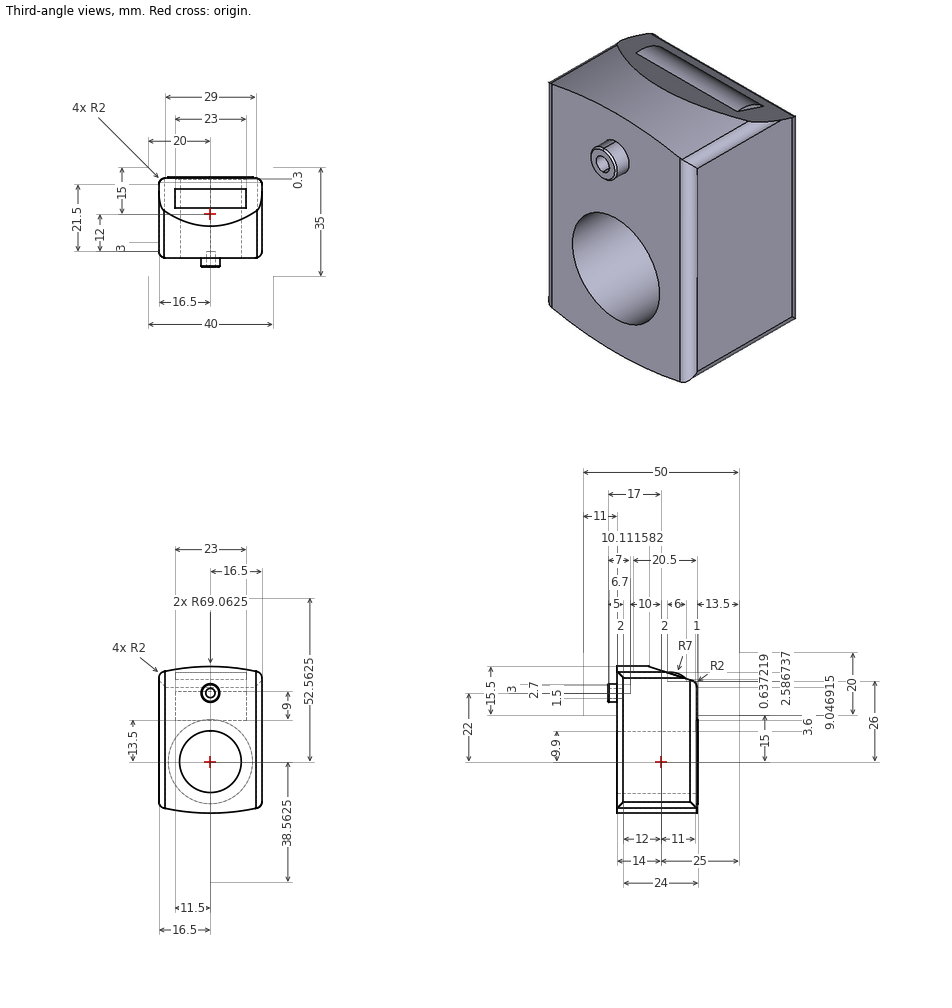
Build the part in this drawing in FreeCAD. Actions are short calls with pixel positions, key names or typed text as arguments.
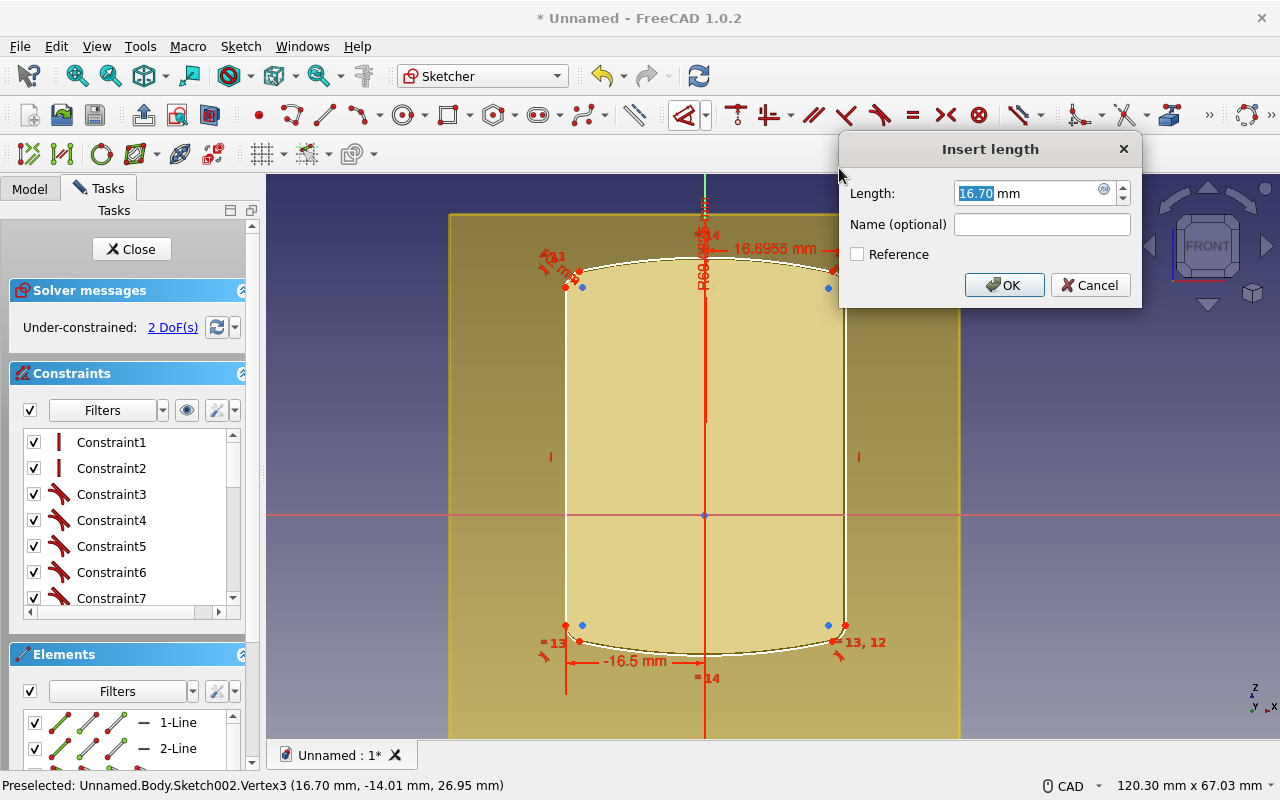
text(16.5)
key(Return)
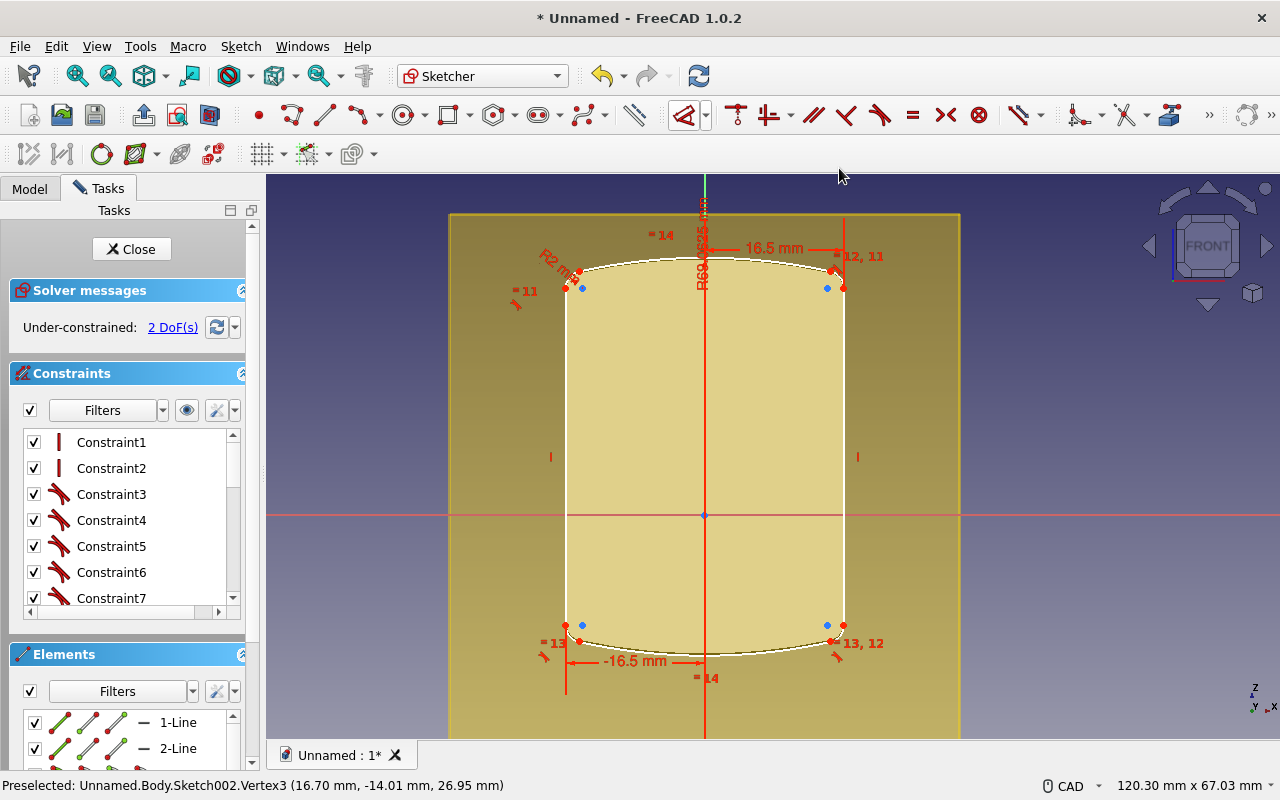
scroll(704, 268, down, 2)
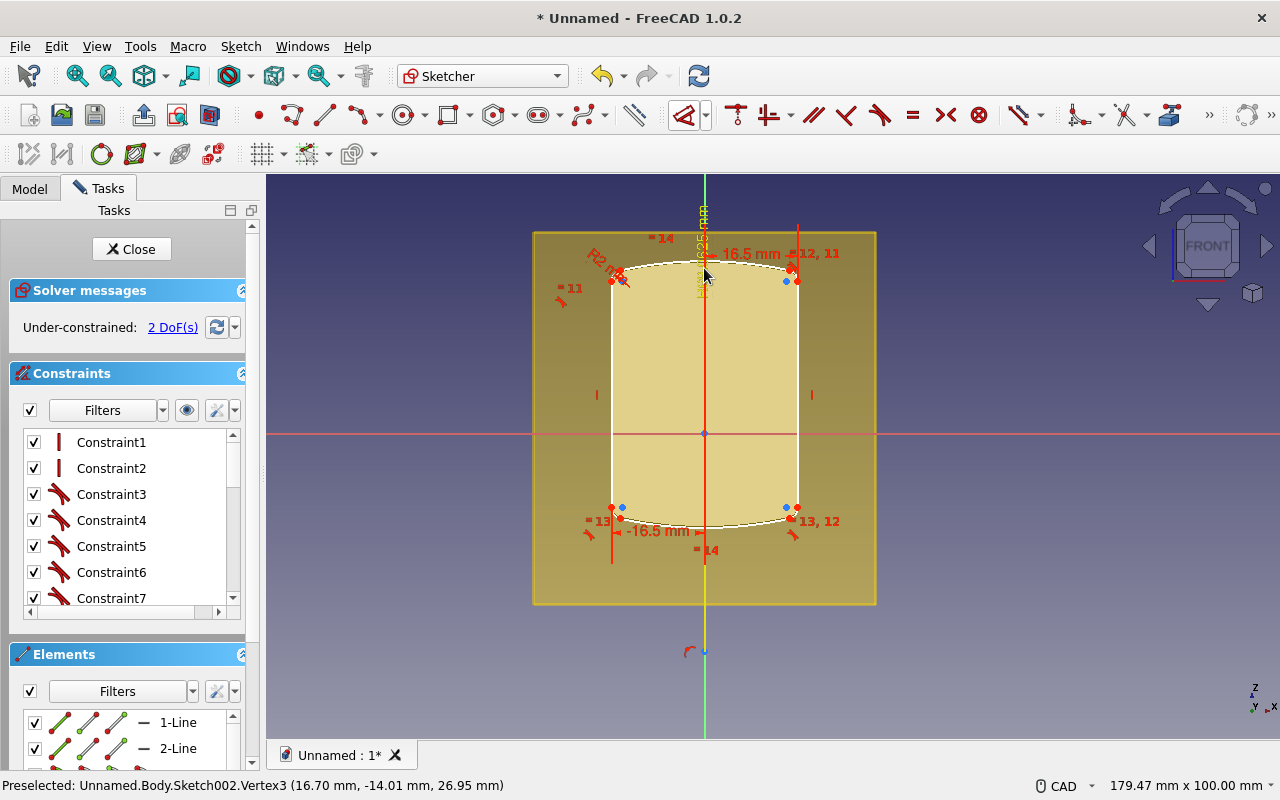
click(705, 651)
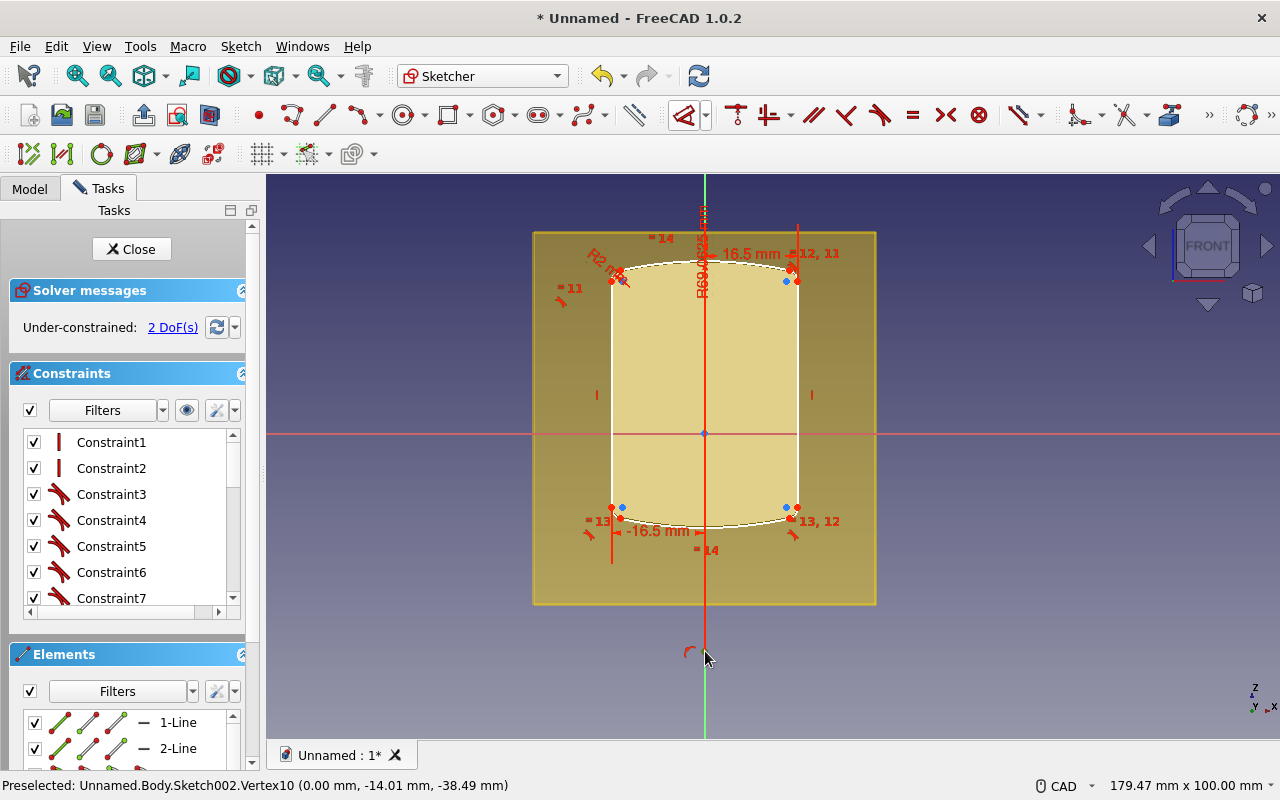
click(706, 116)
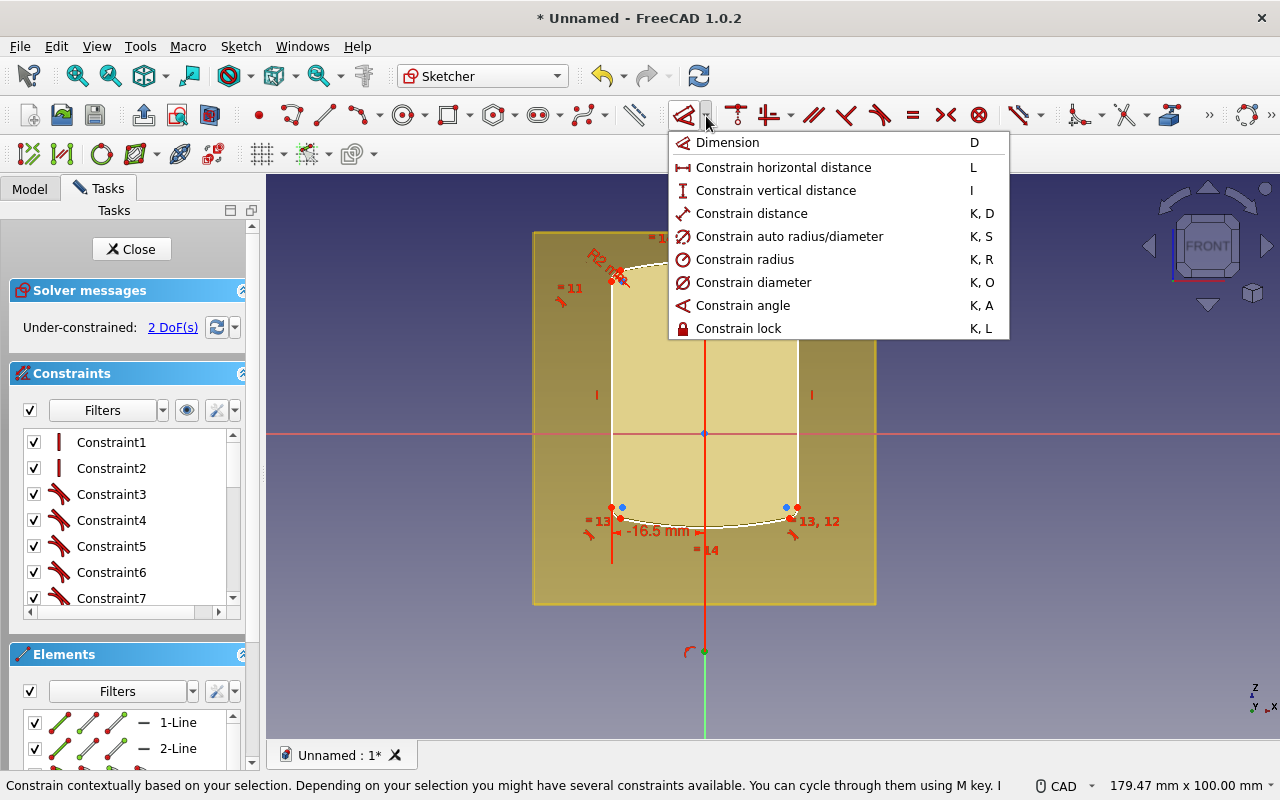
click(839, 190)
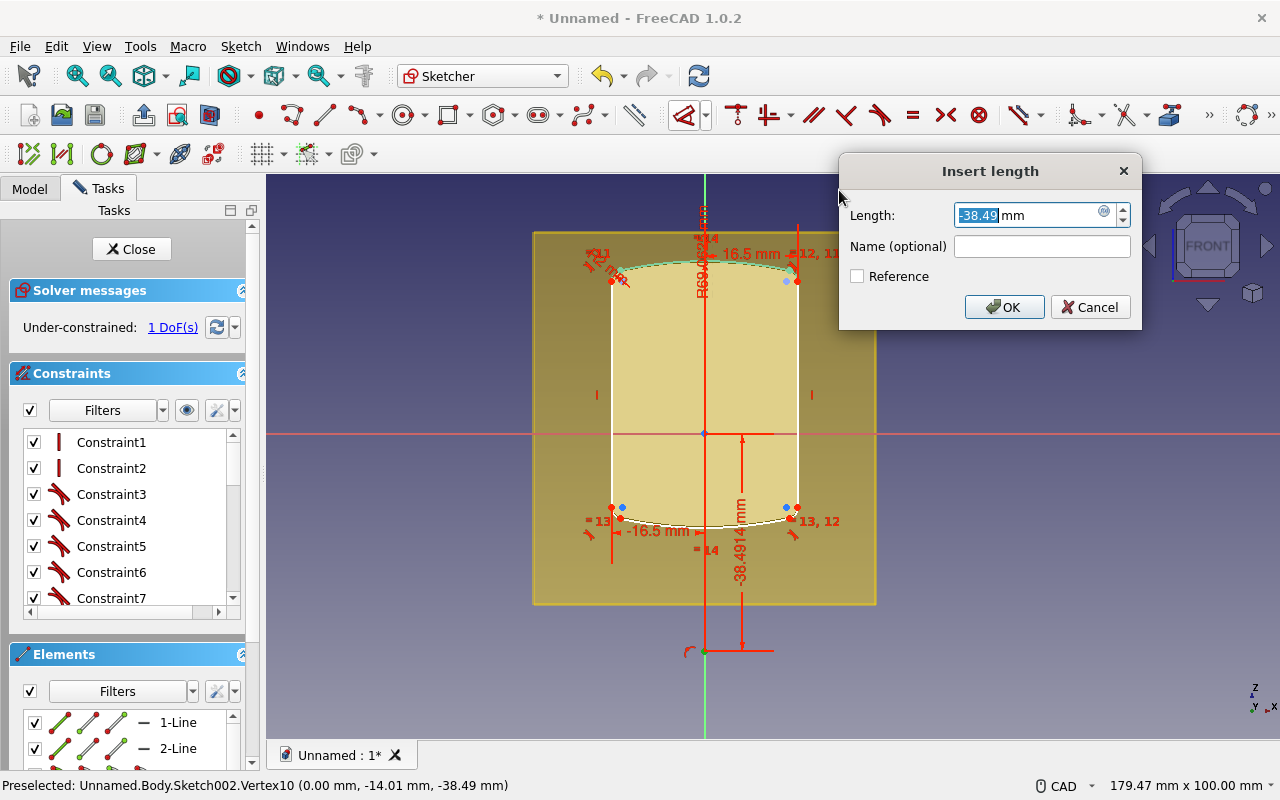
text(-38.5625)
key(Return)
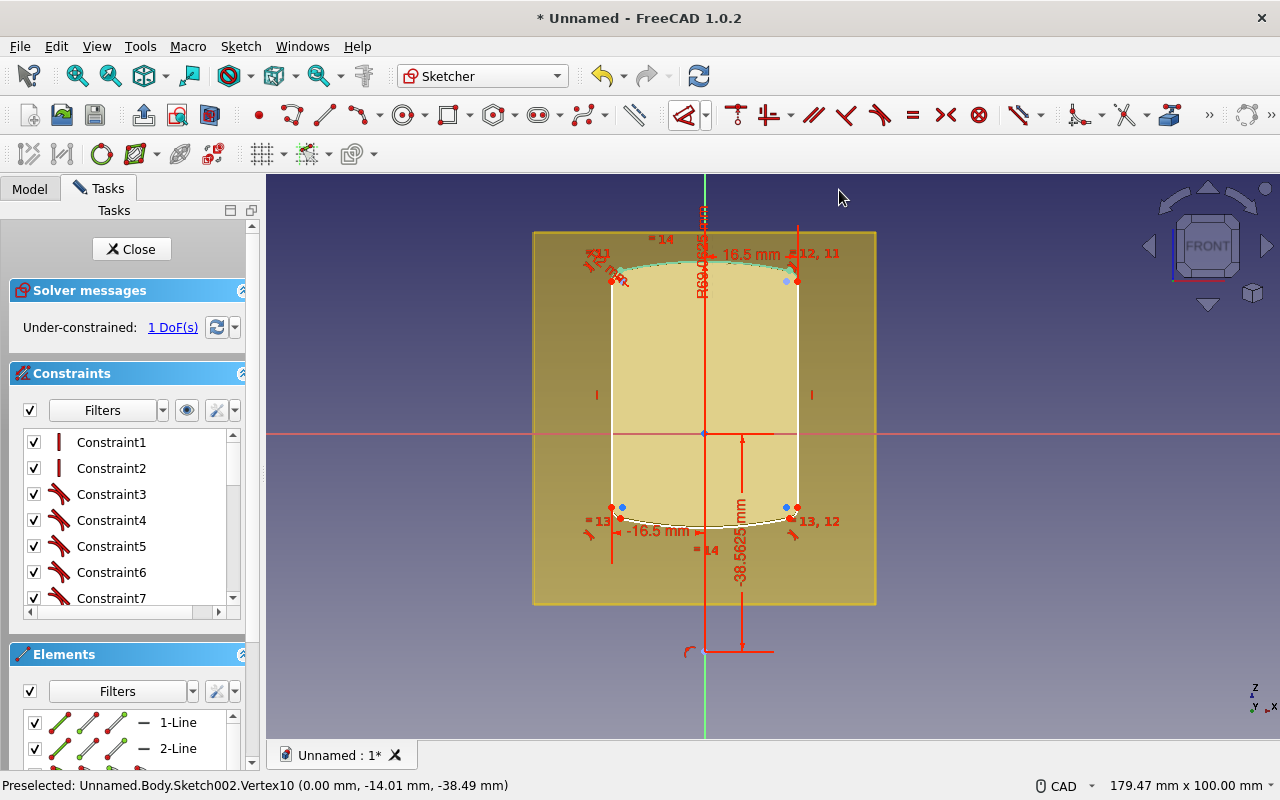
scroll(705, 268, up, 2)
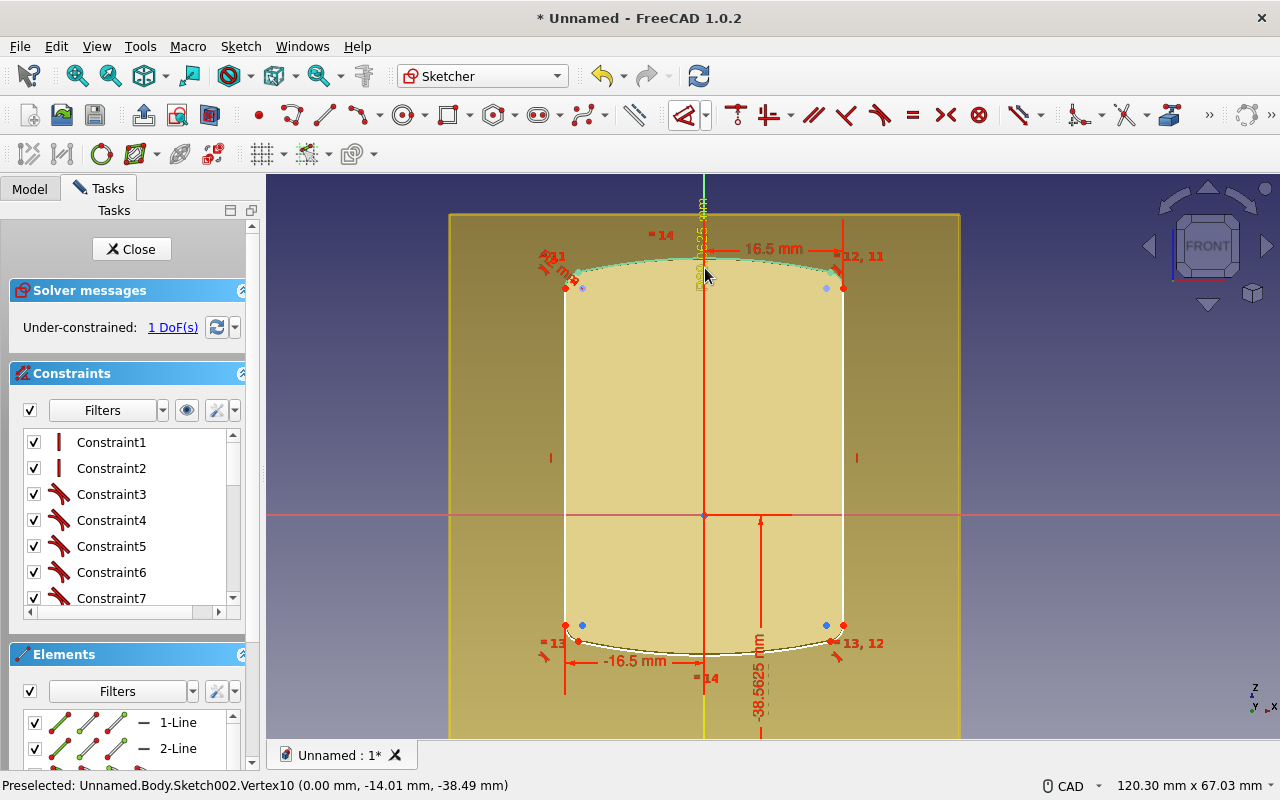
scroll(705, 644, down, 2)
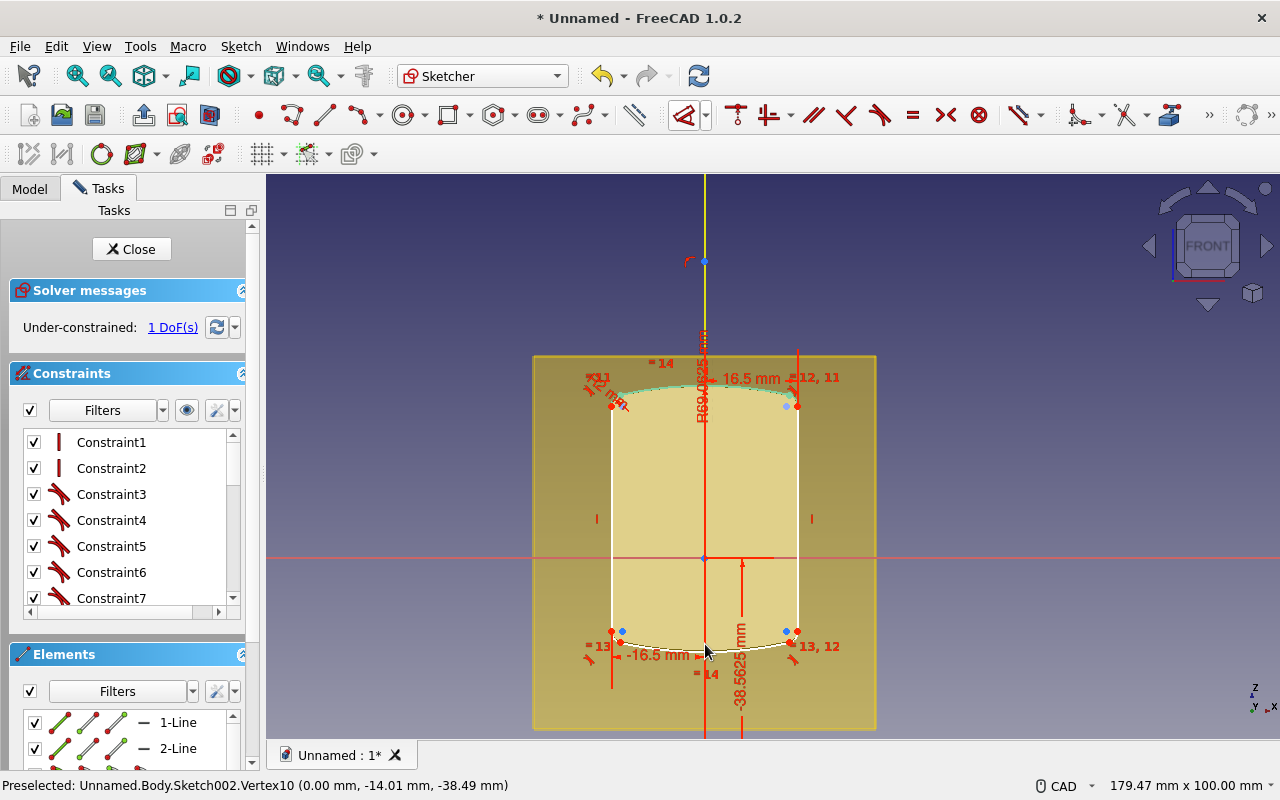
click(705, 262)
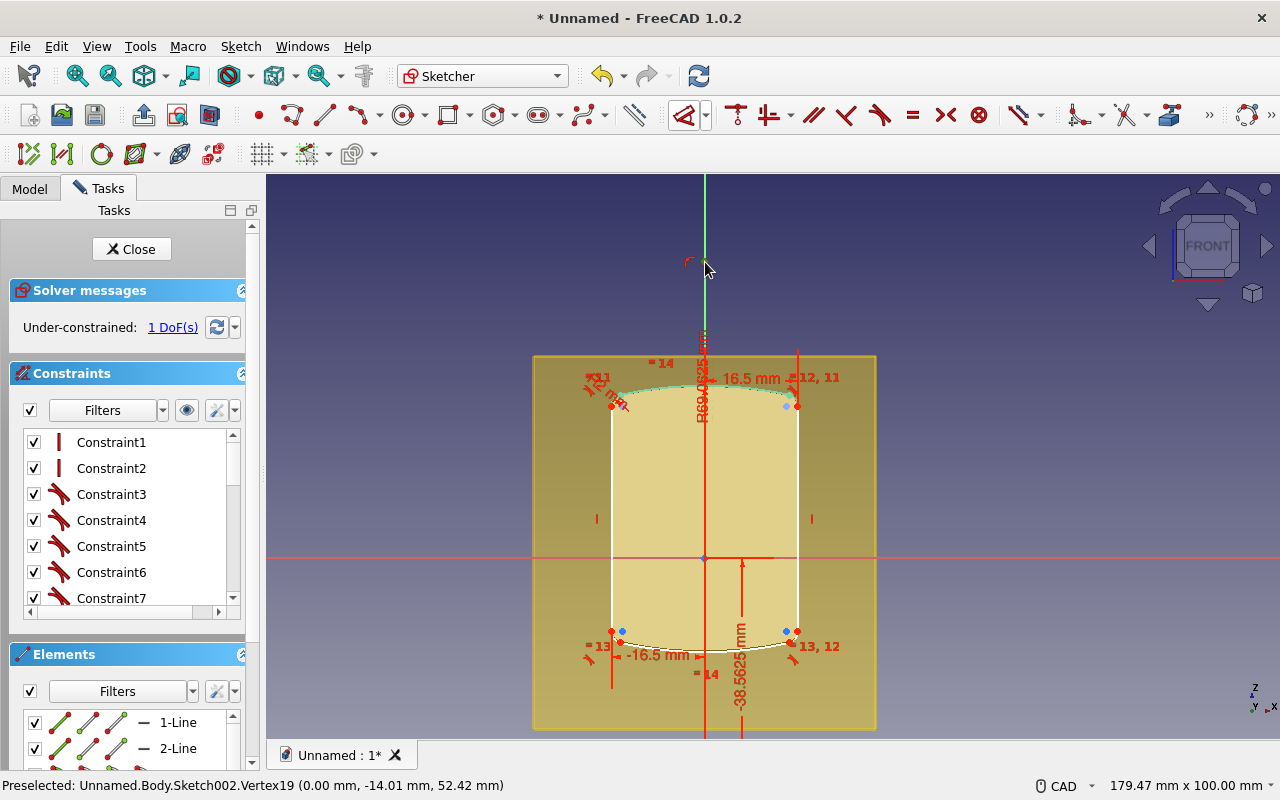
key(i)